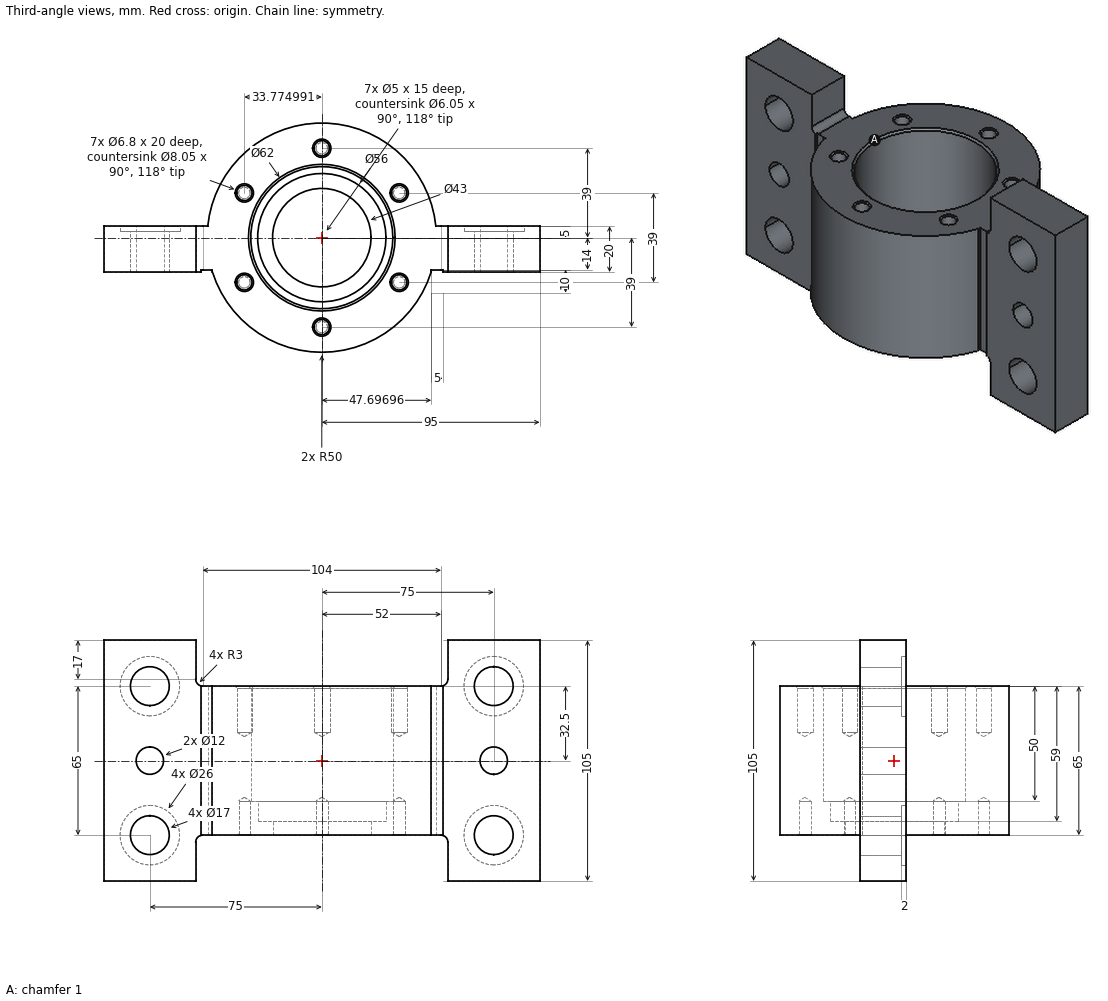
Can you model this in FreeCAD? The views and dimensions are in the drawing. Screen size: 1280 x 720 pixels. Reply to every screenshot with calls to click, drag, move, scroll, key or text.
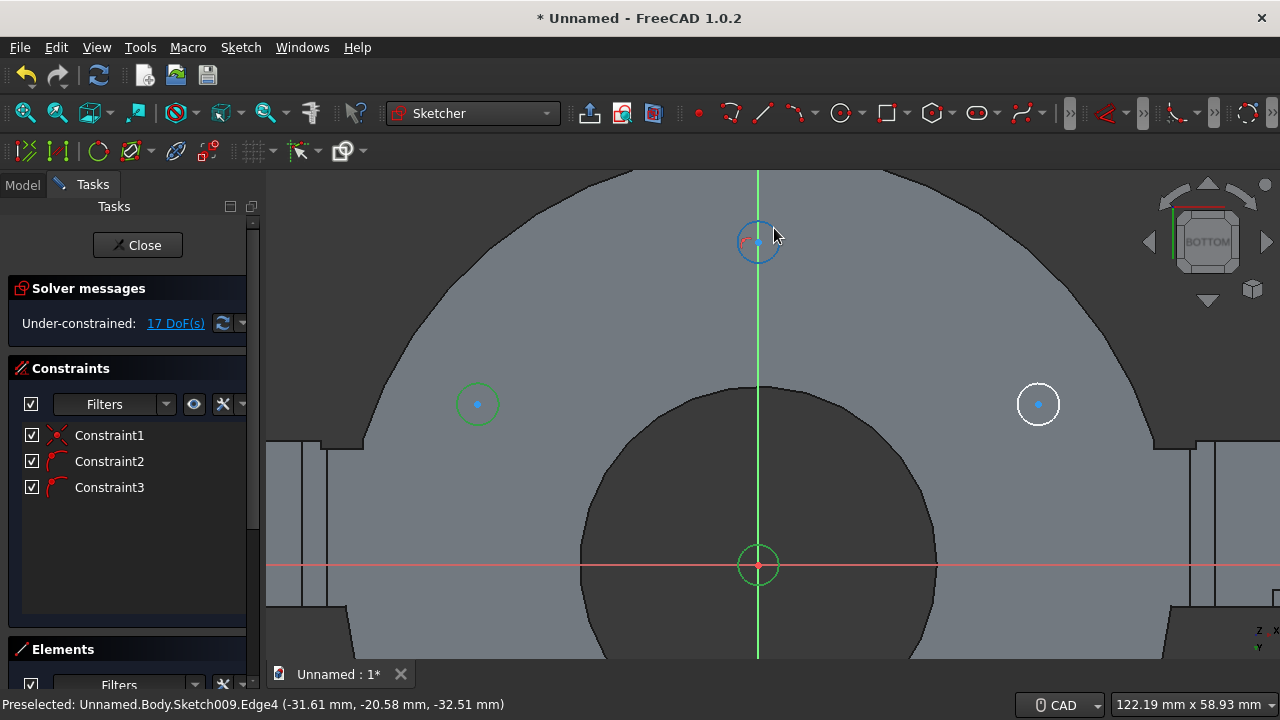
click(773, 227)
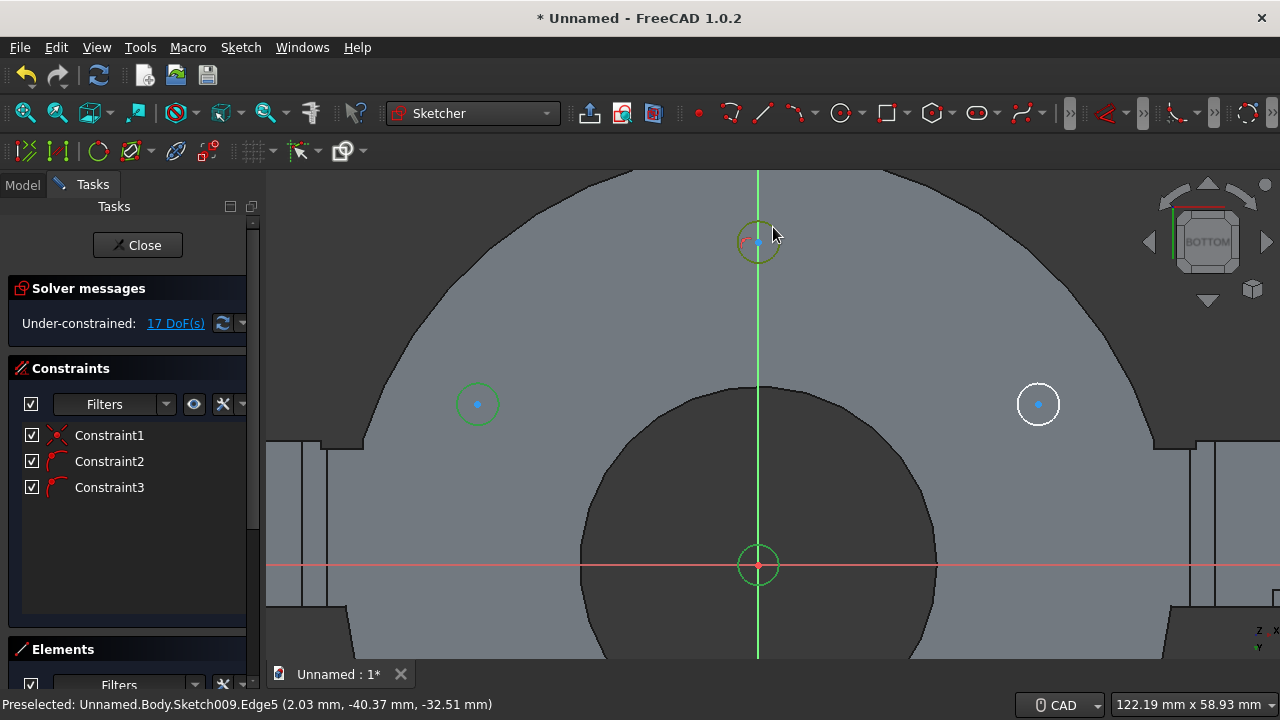
click(1053, 390)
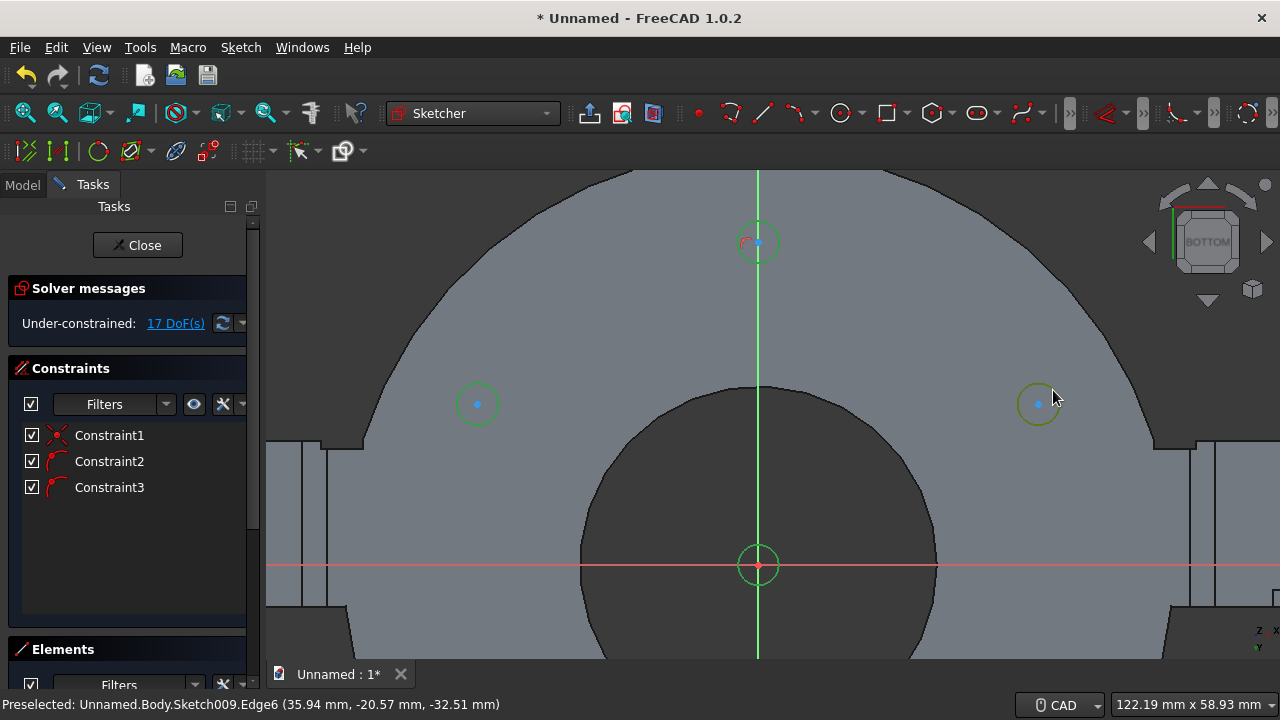
scroll(660, 292, down, 4)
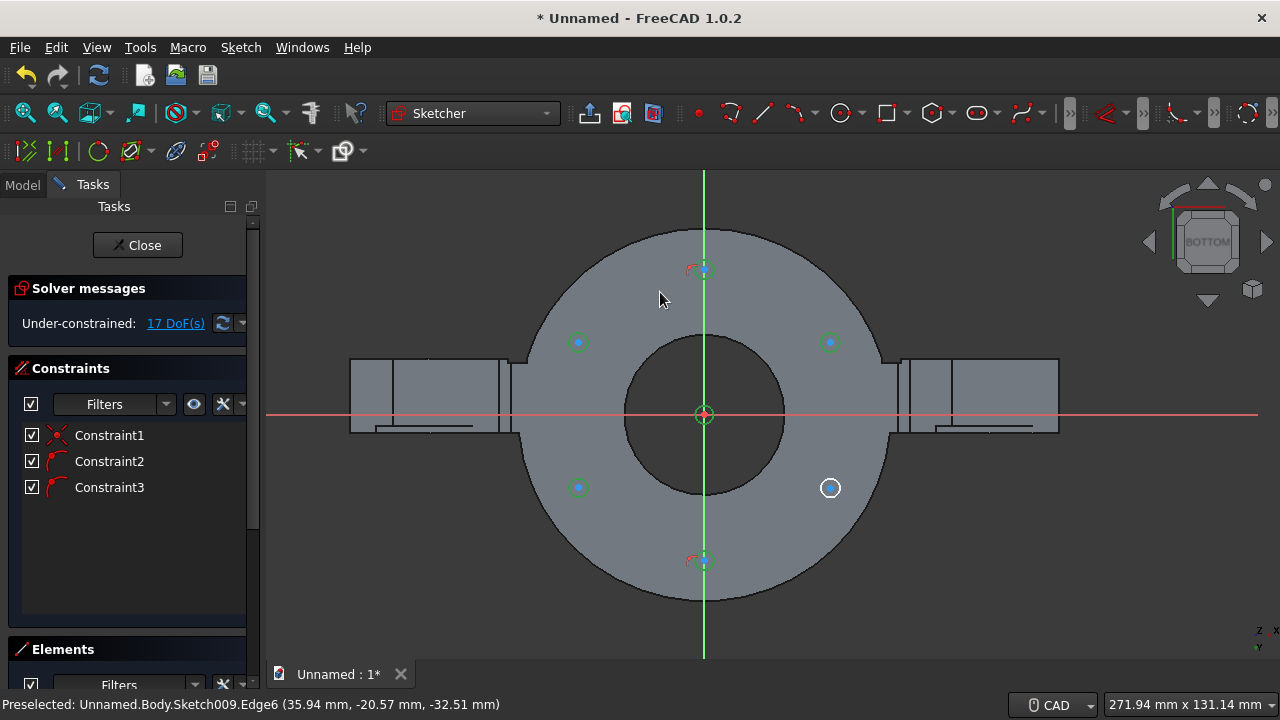
scroll(837, 481, up, 2)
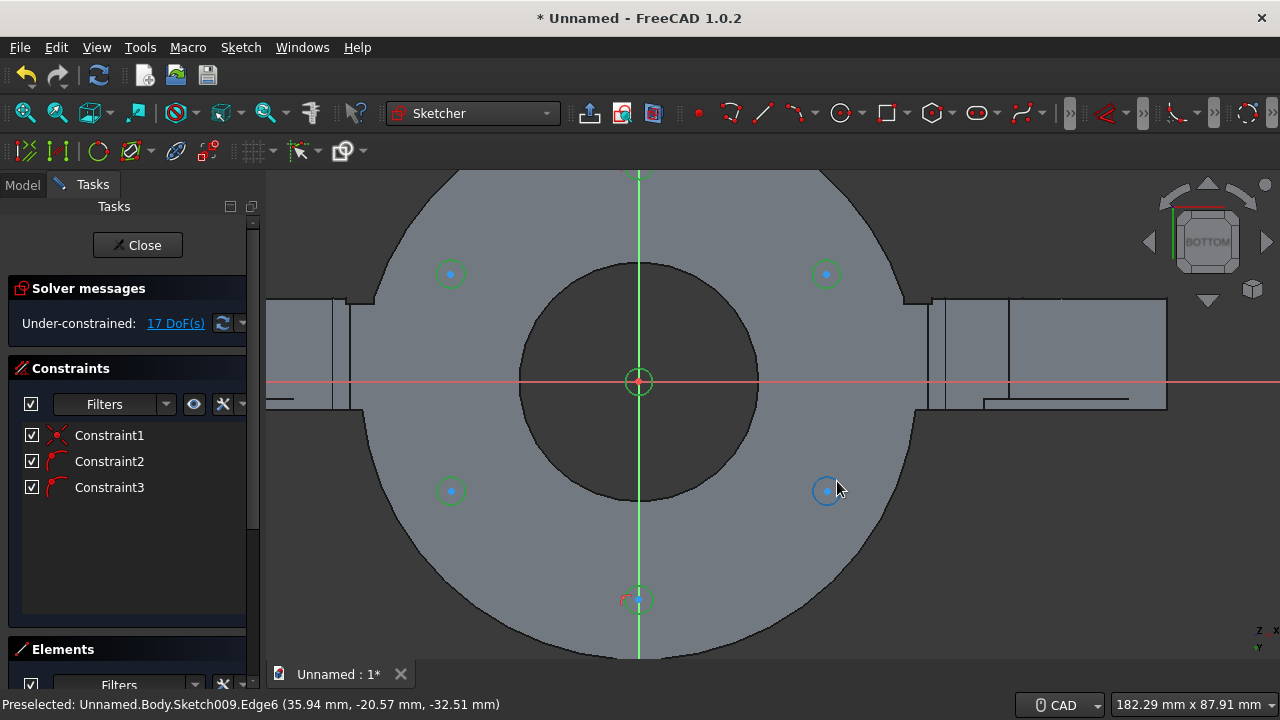
click(837, 481)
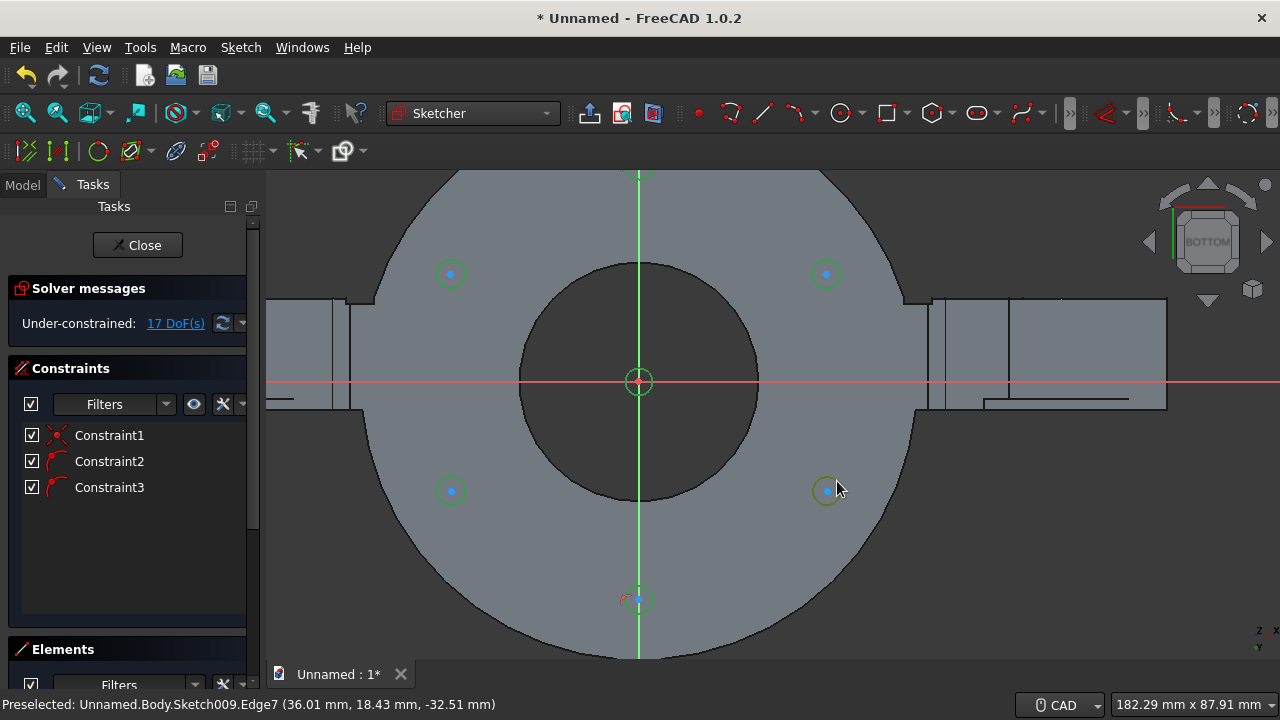
key(e)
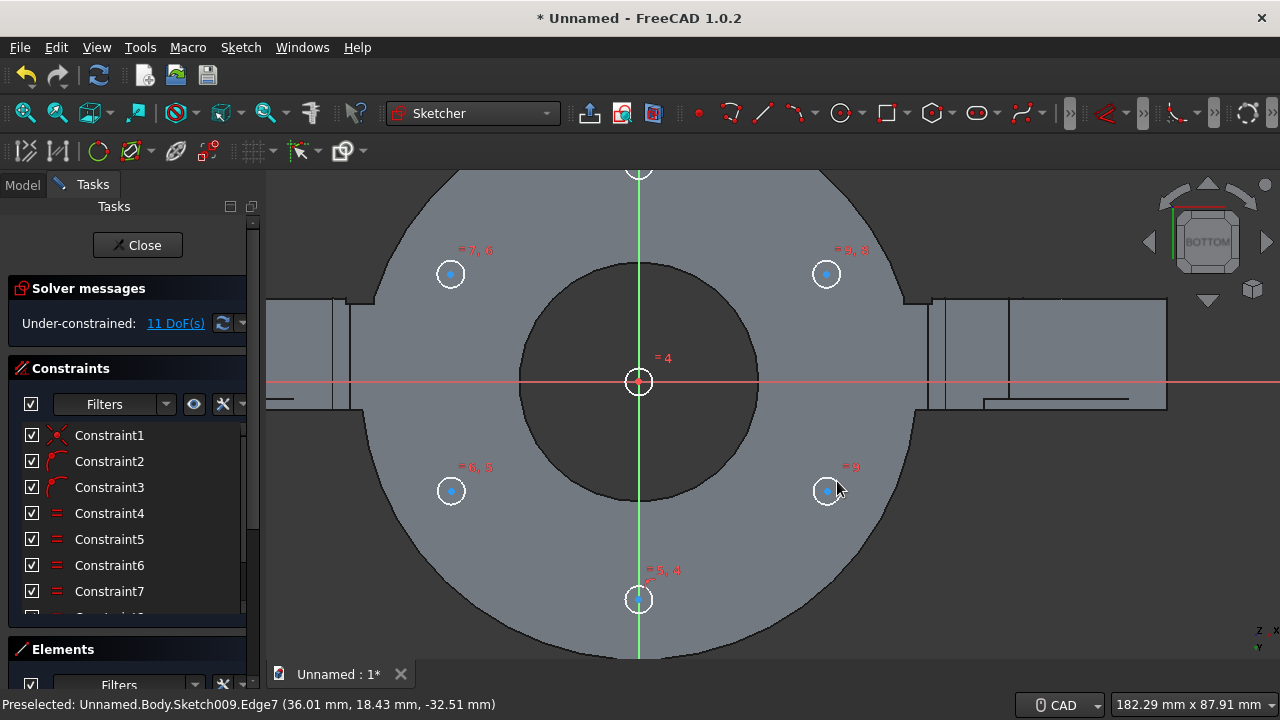
click(451, 491)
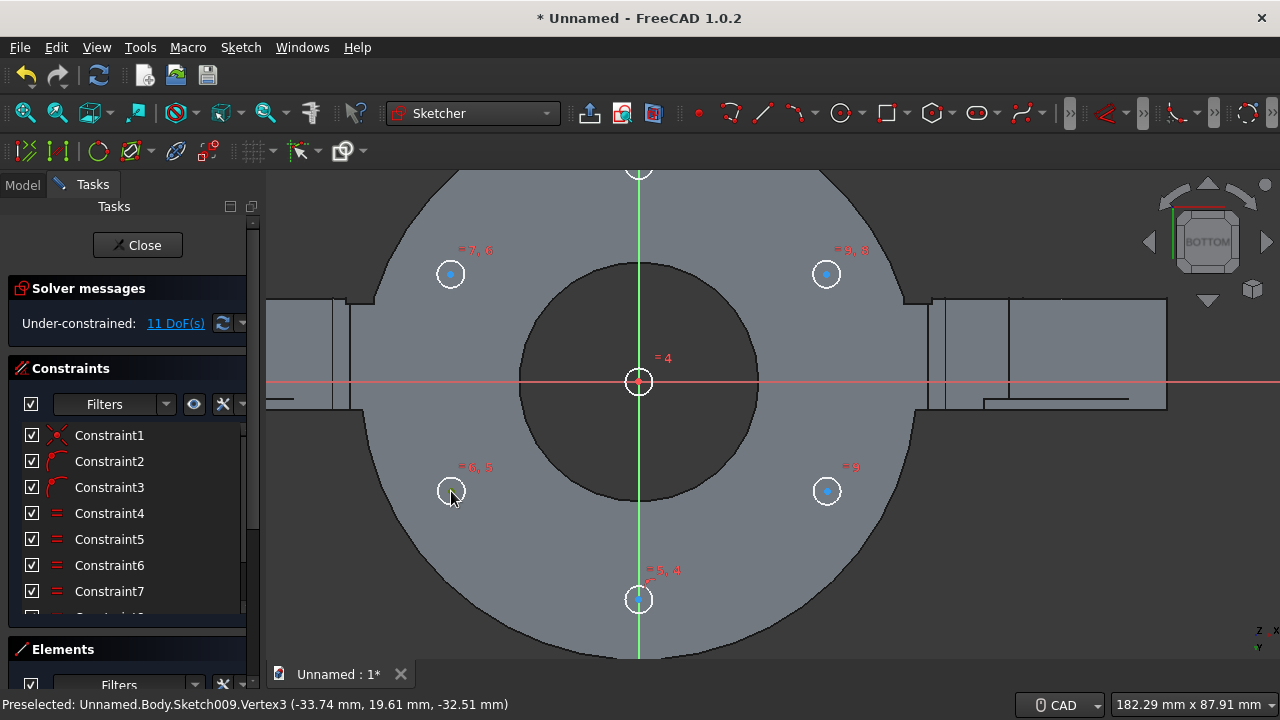
click(451, 274)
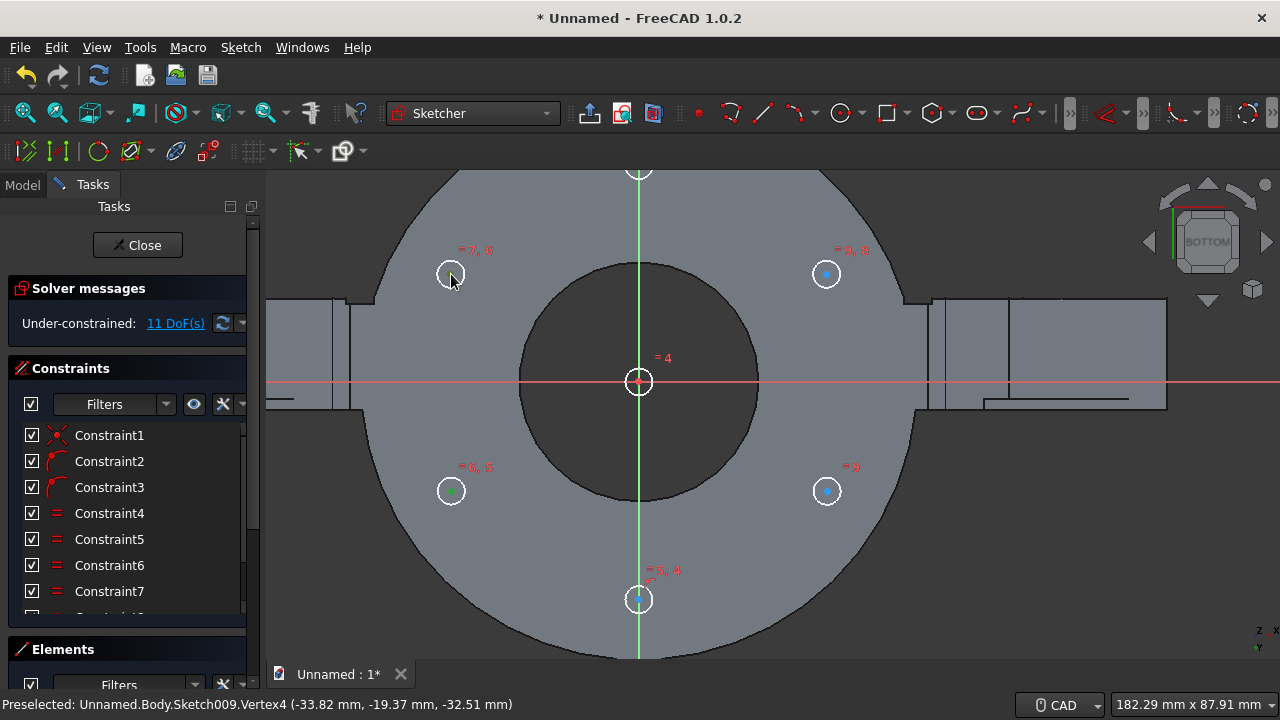
click(353, 382)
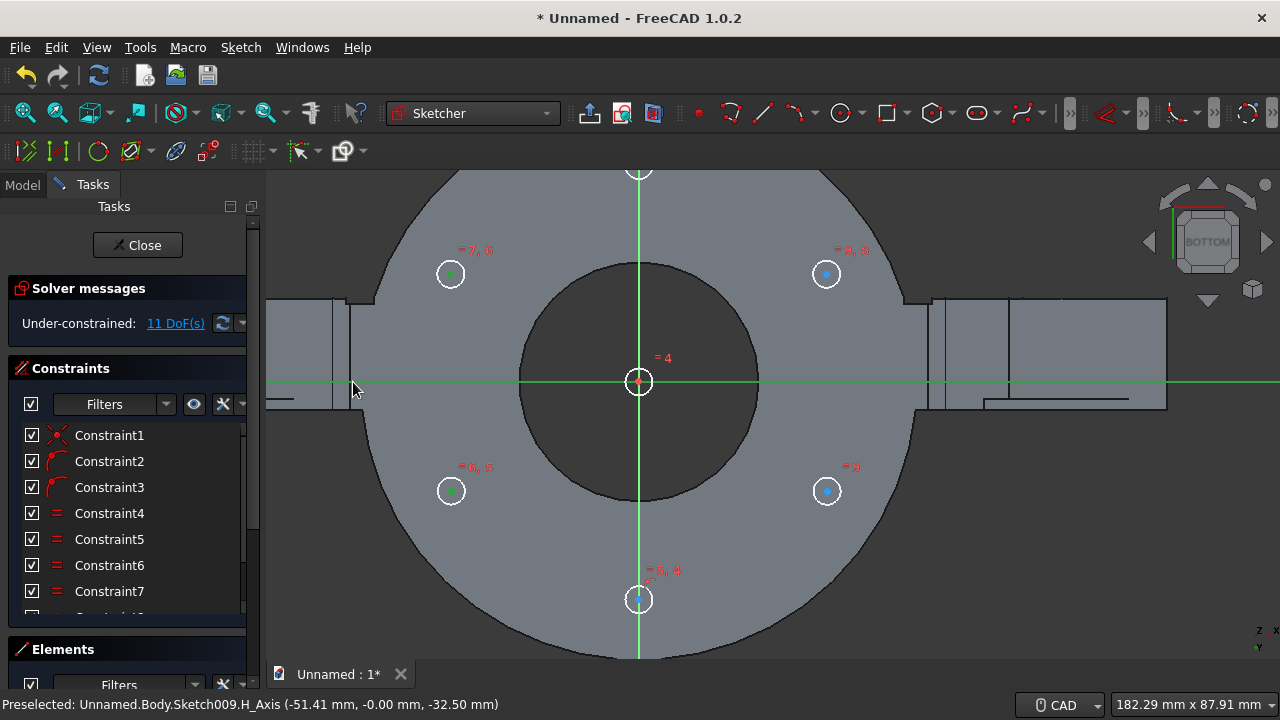
key(s)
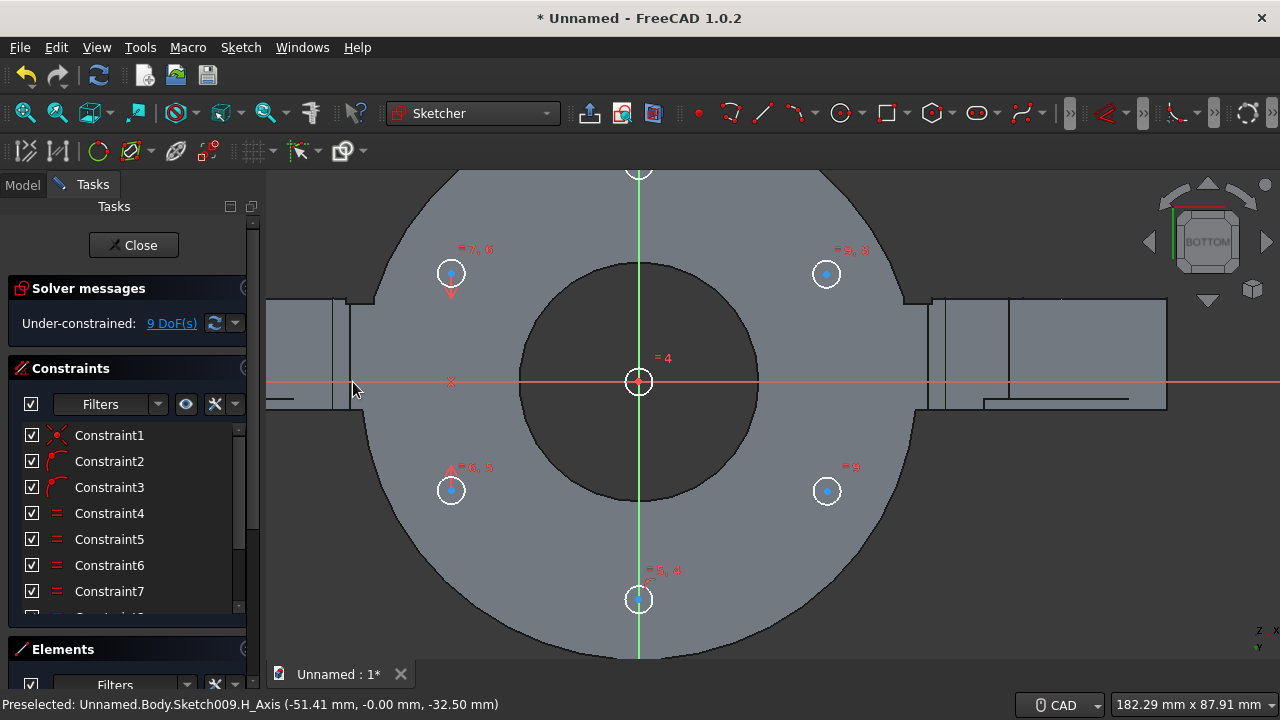
click(451, 273)